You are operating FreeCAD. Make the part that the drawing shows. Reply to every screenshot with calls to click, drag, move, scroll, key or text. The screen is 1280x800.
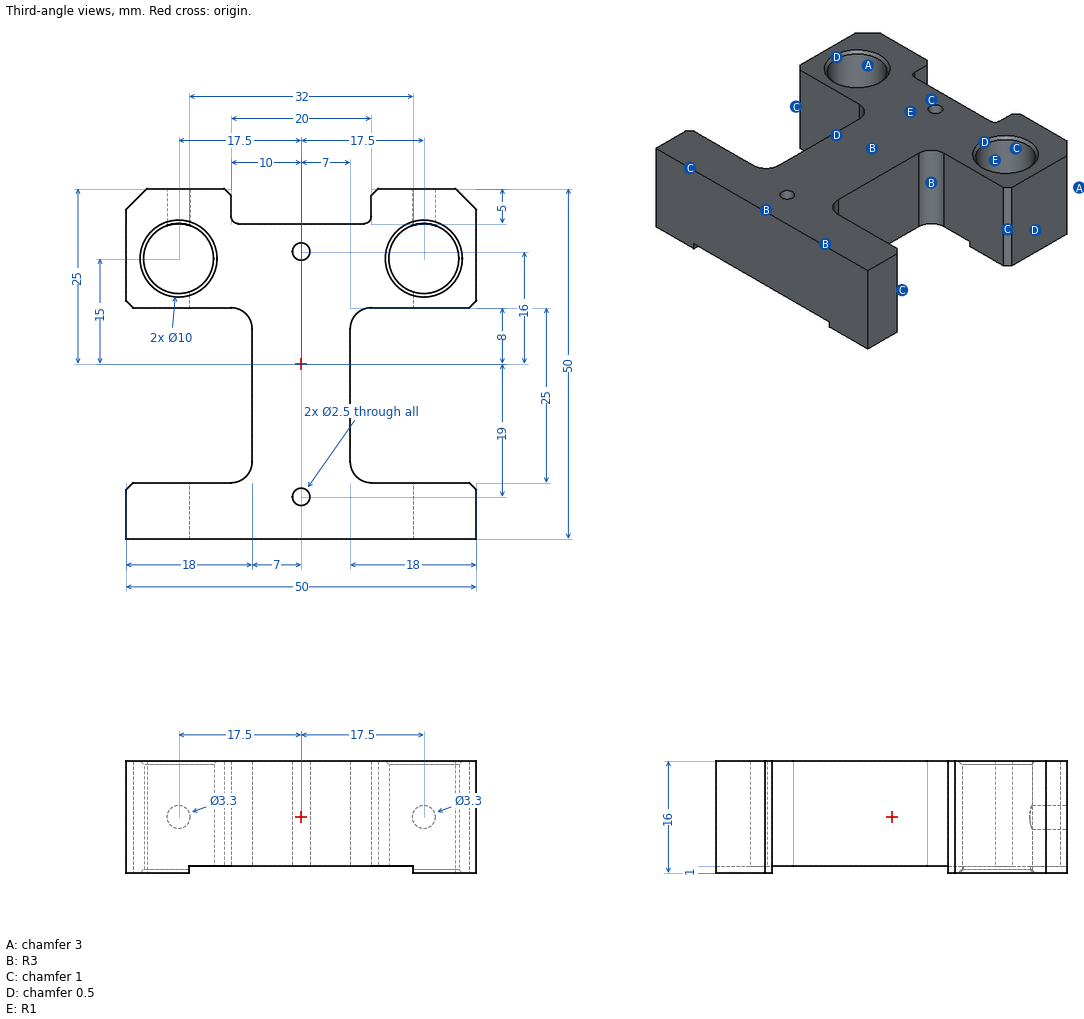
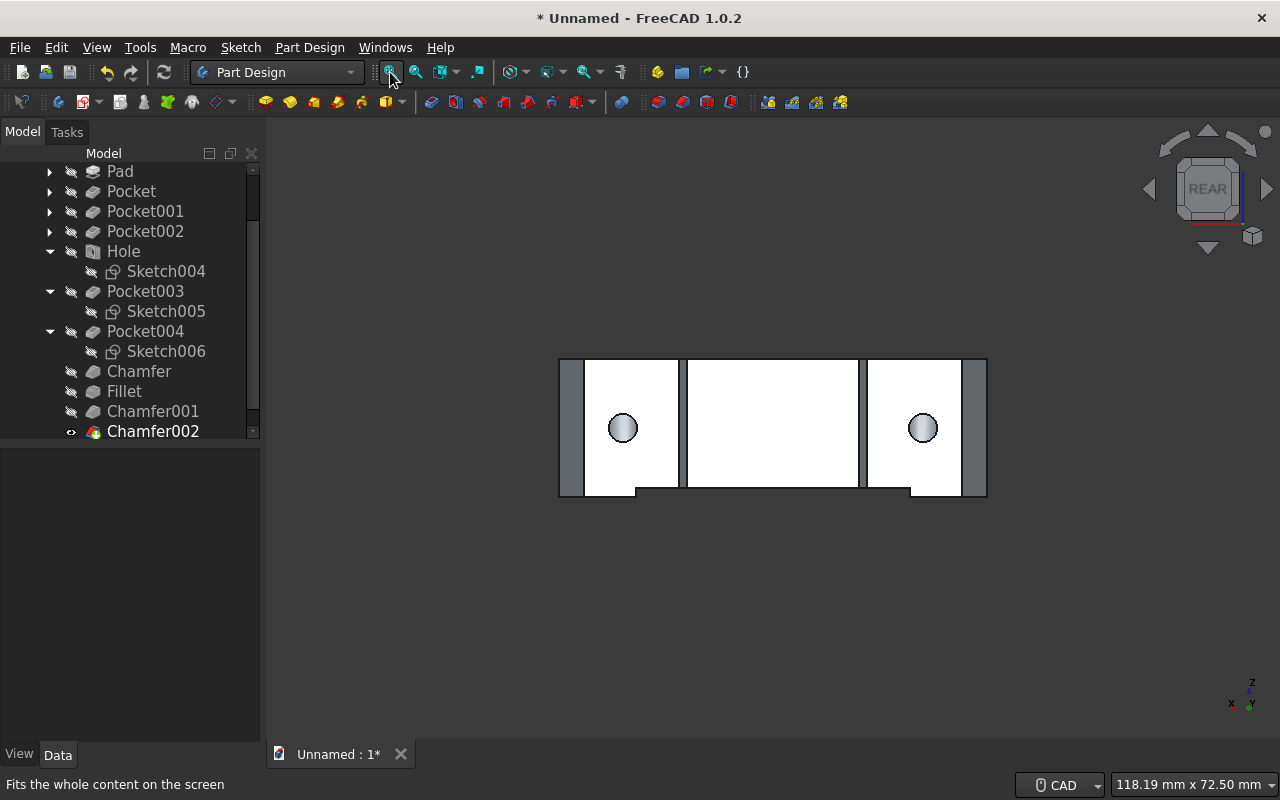
key(6)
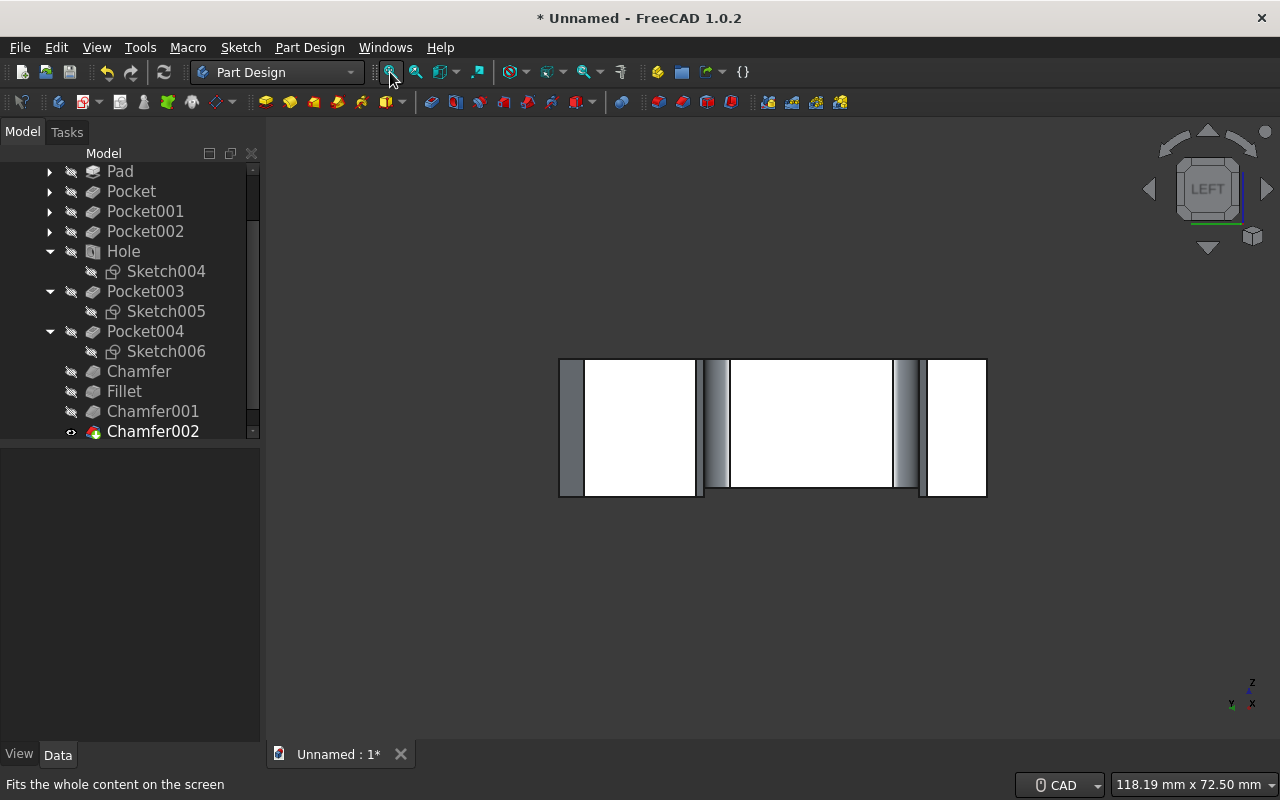
key(v)
key(f)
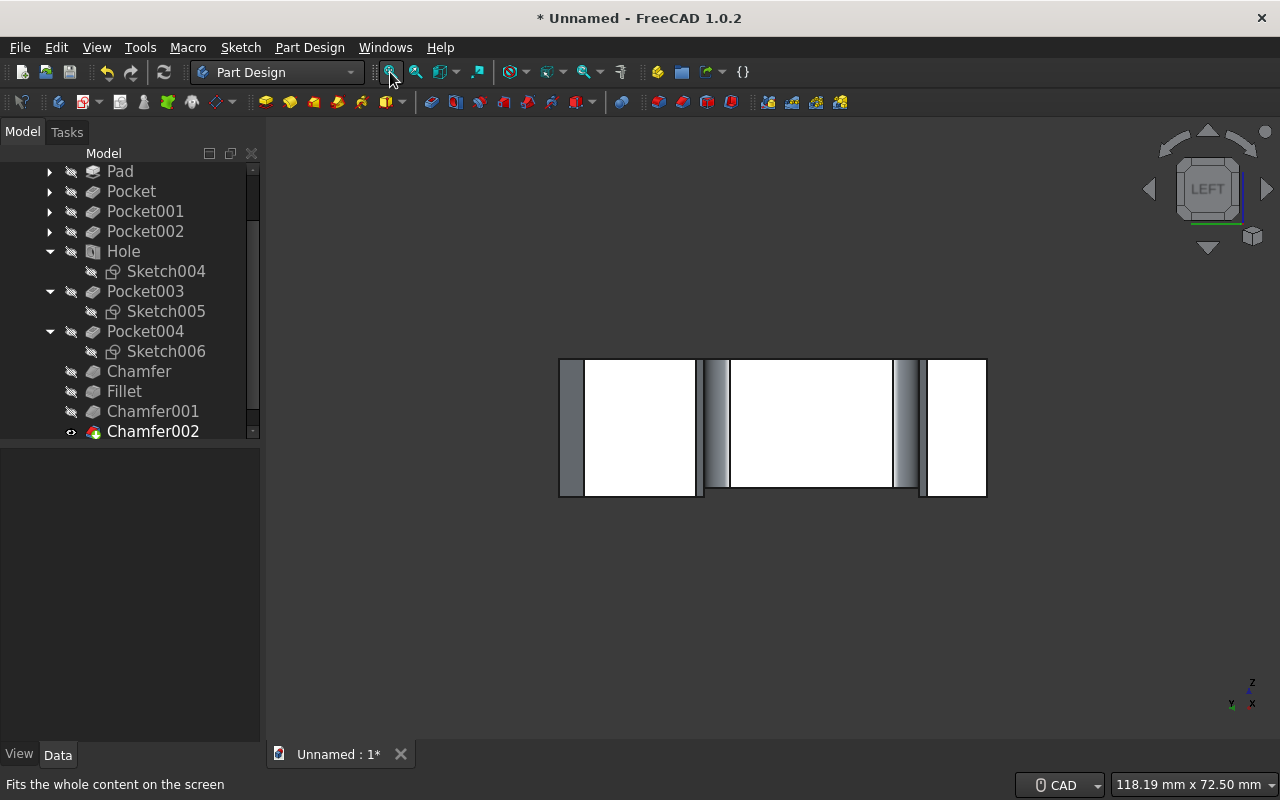
key(v)
key(3)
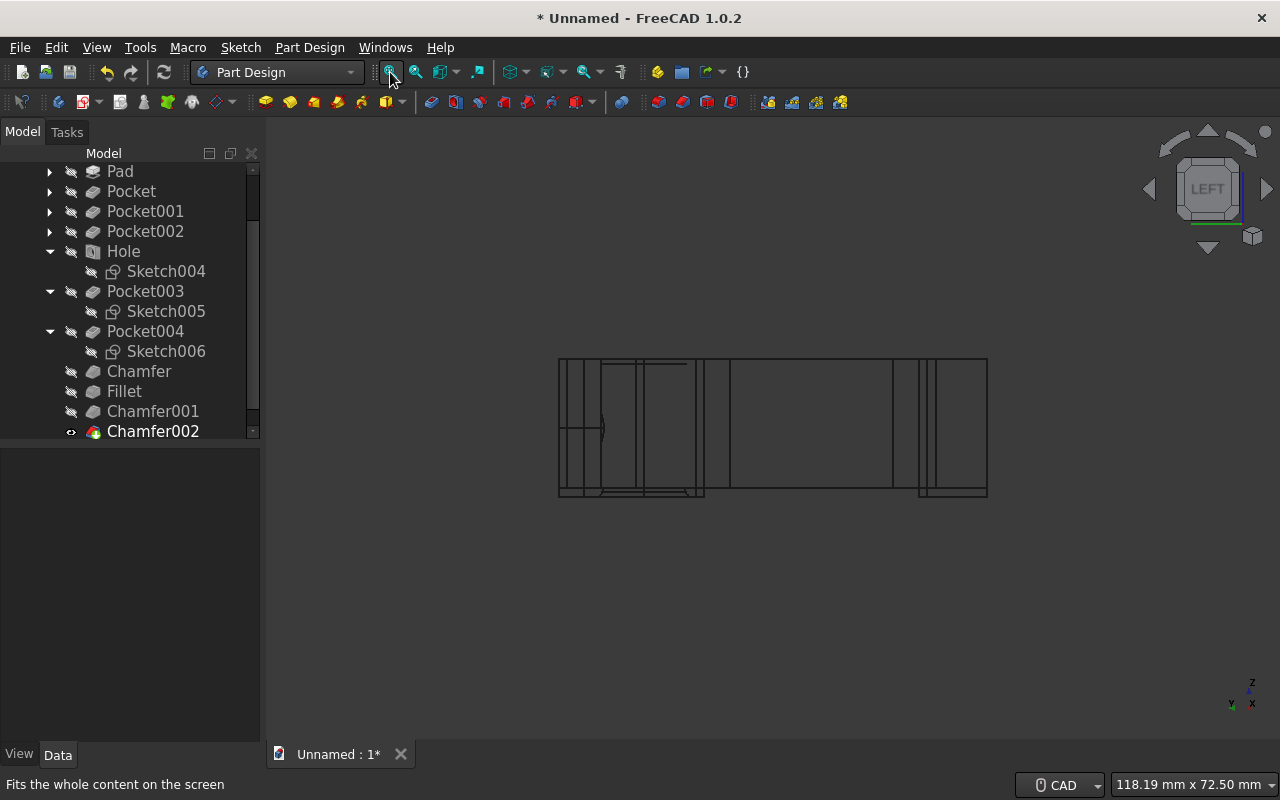
key(0)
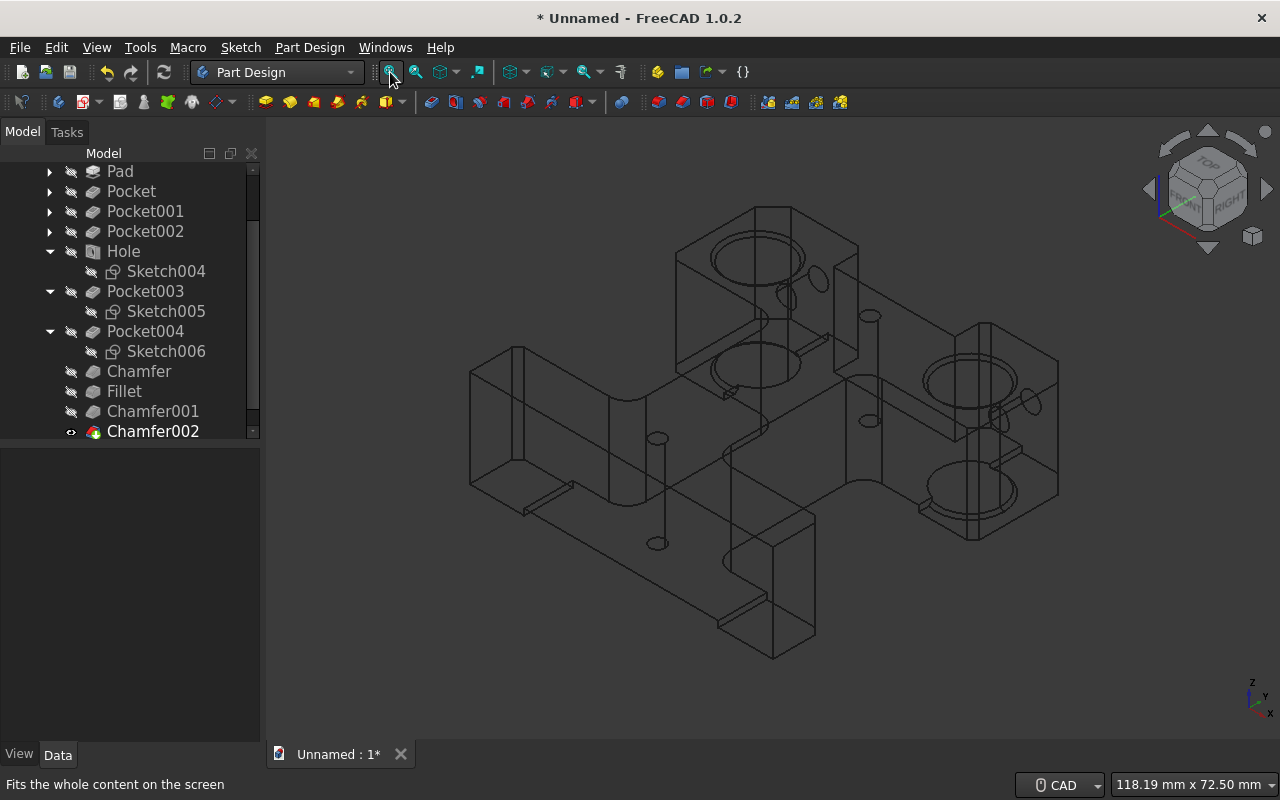
click(834, 318)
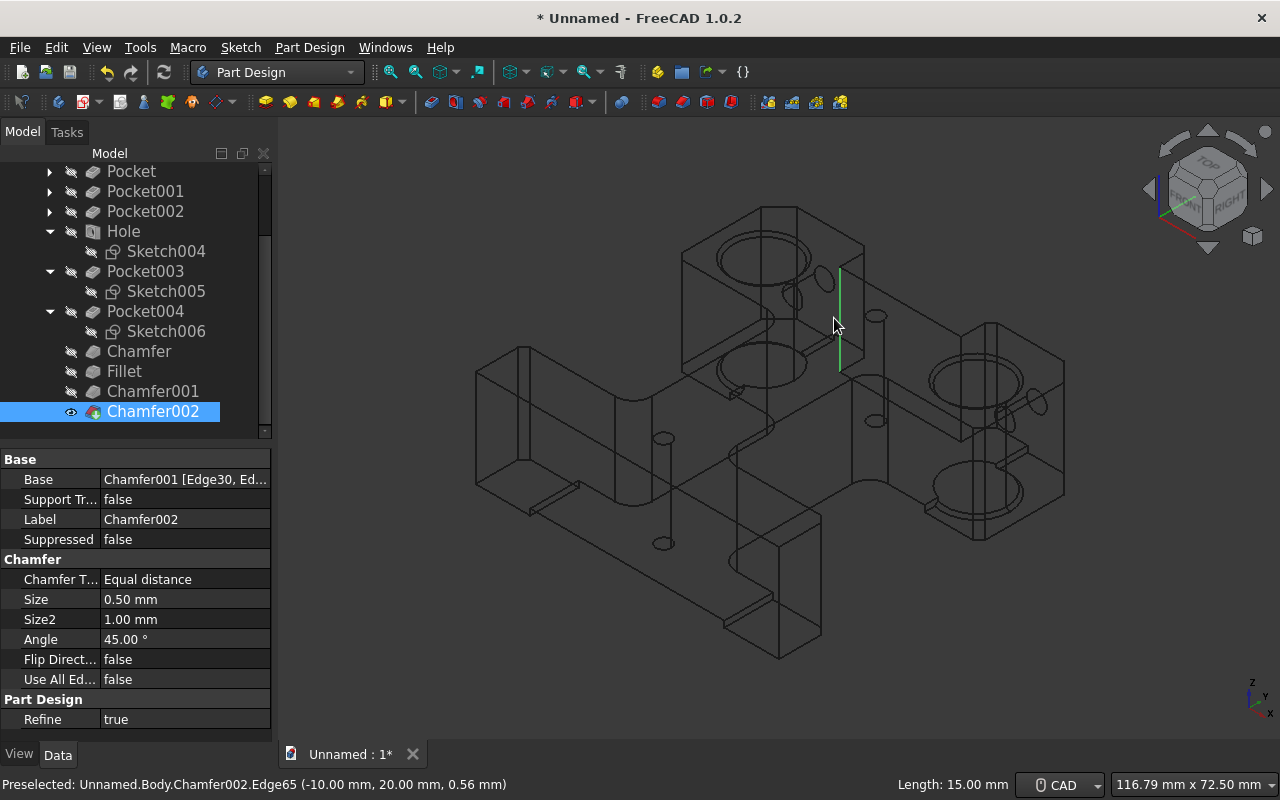
click(961, 388, ctrl)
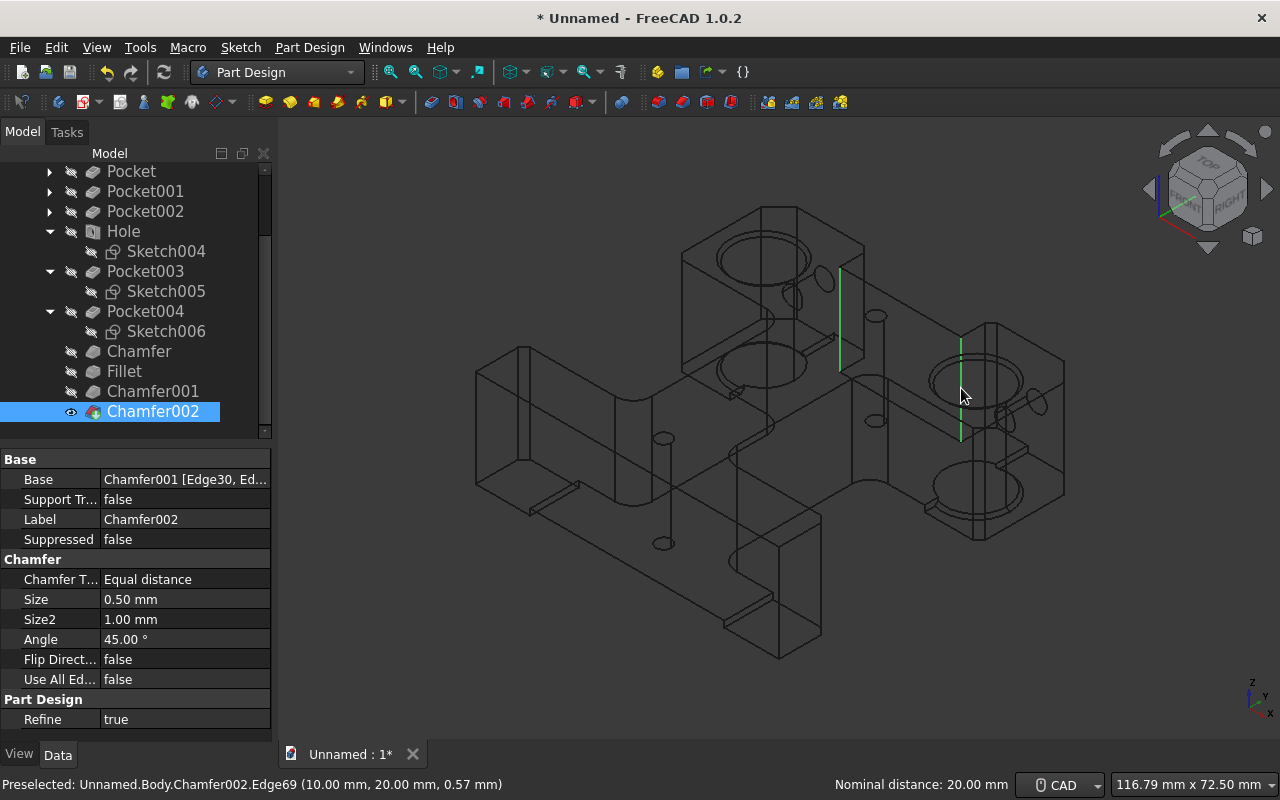
key(v)
key(1)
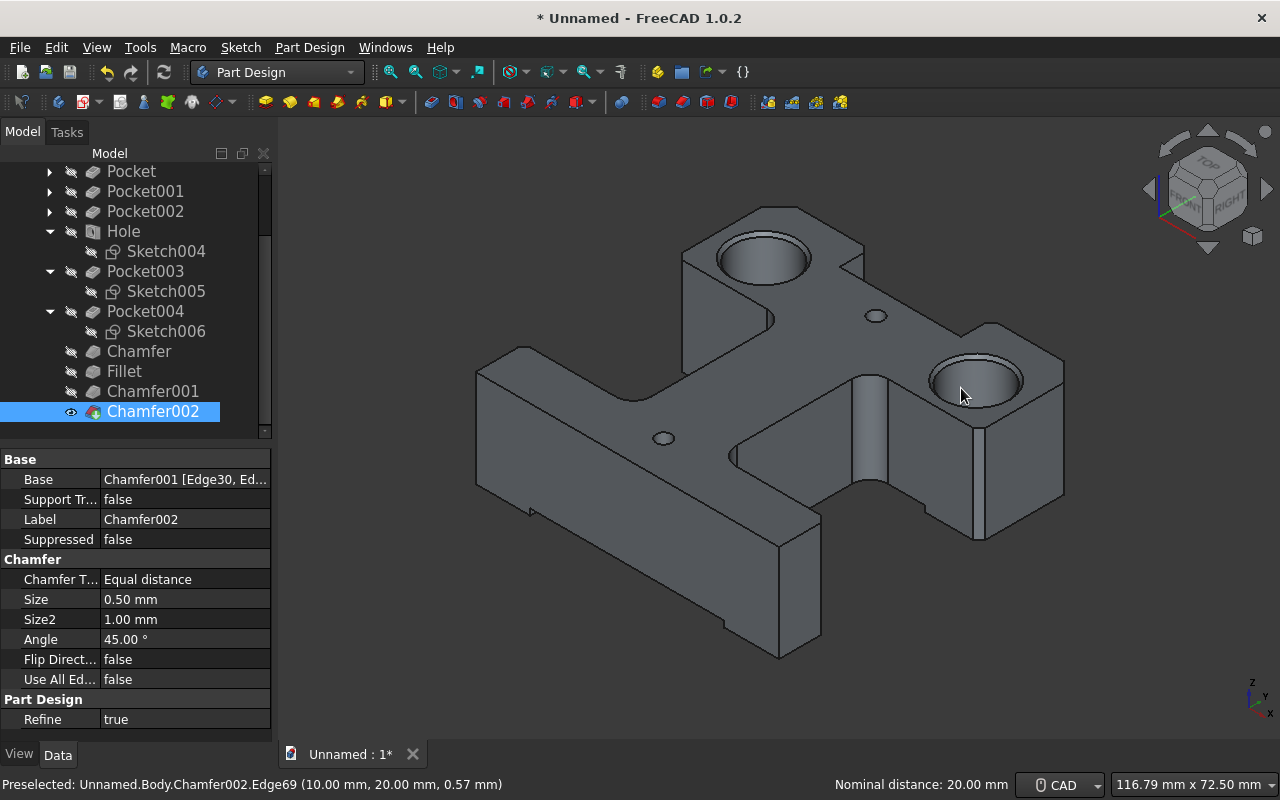
click(660, 102)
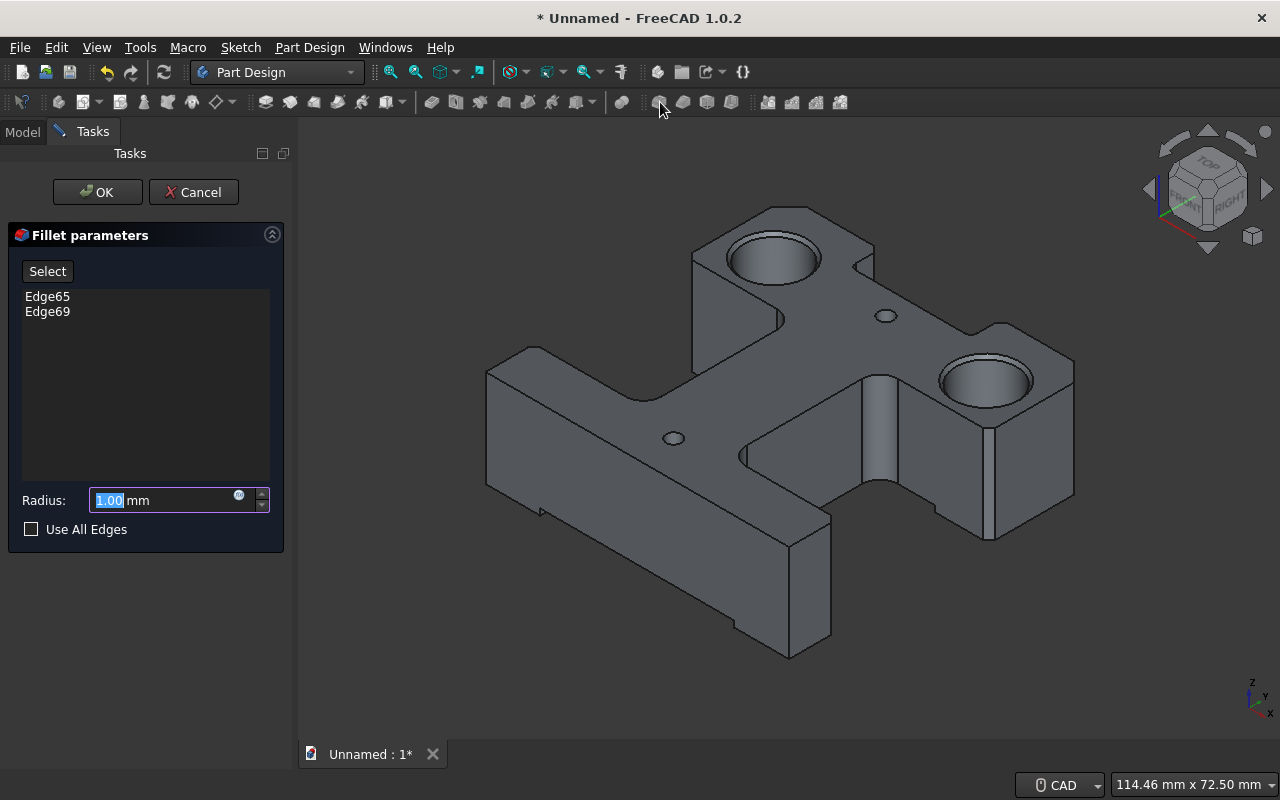
text(1)
key(Tab)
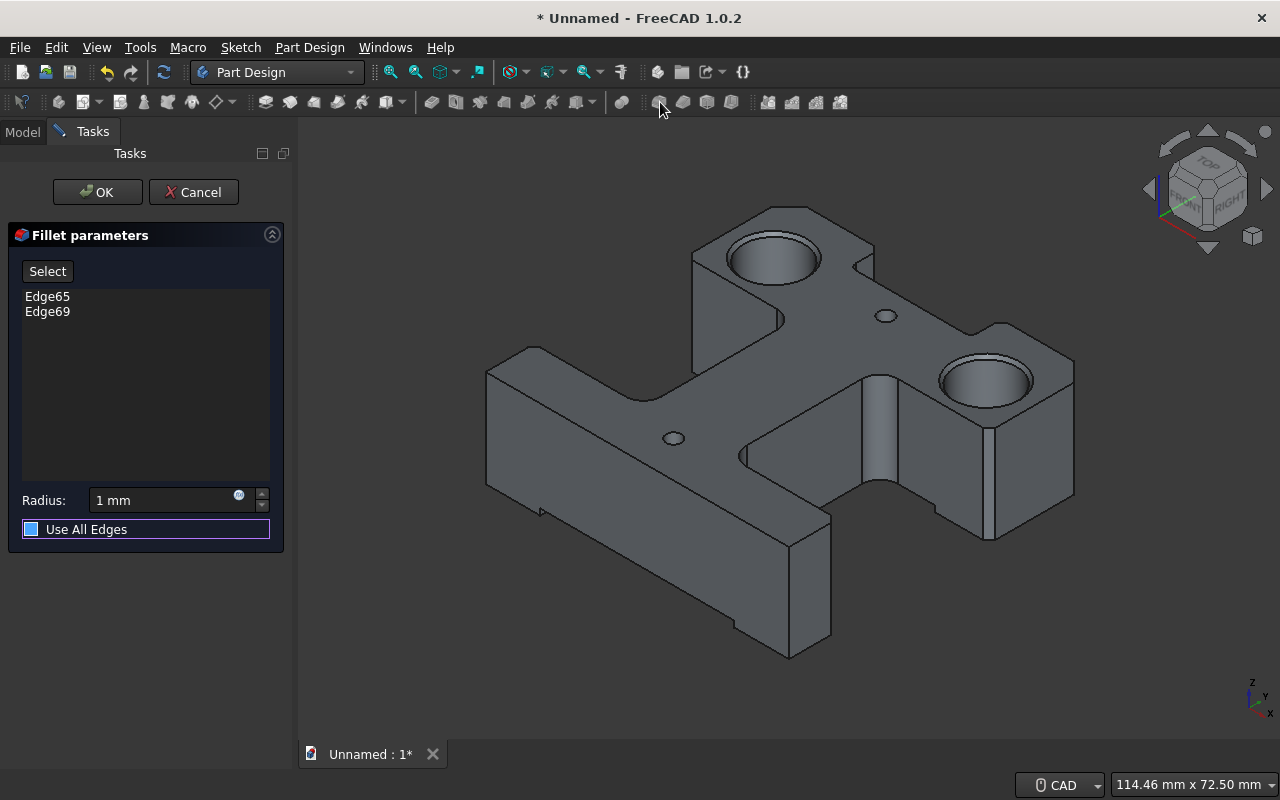
click(98, 192)